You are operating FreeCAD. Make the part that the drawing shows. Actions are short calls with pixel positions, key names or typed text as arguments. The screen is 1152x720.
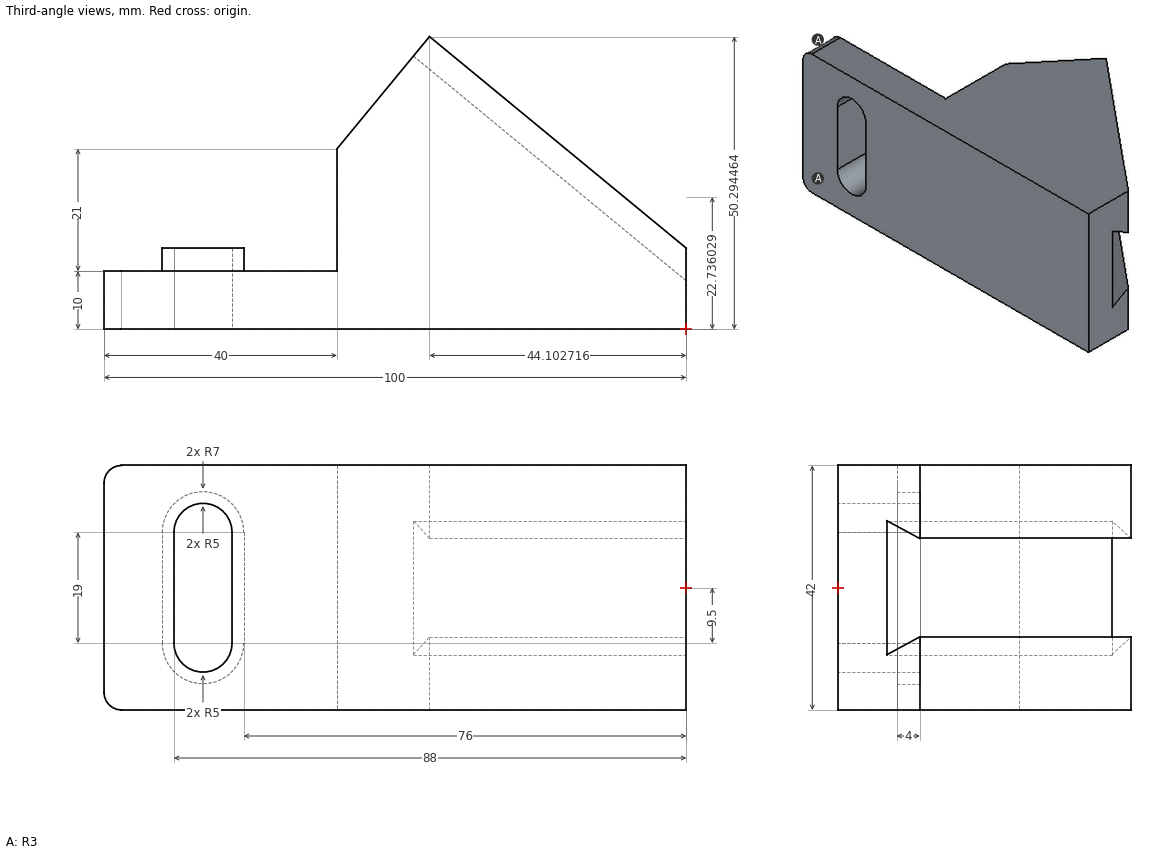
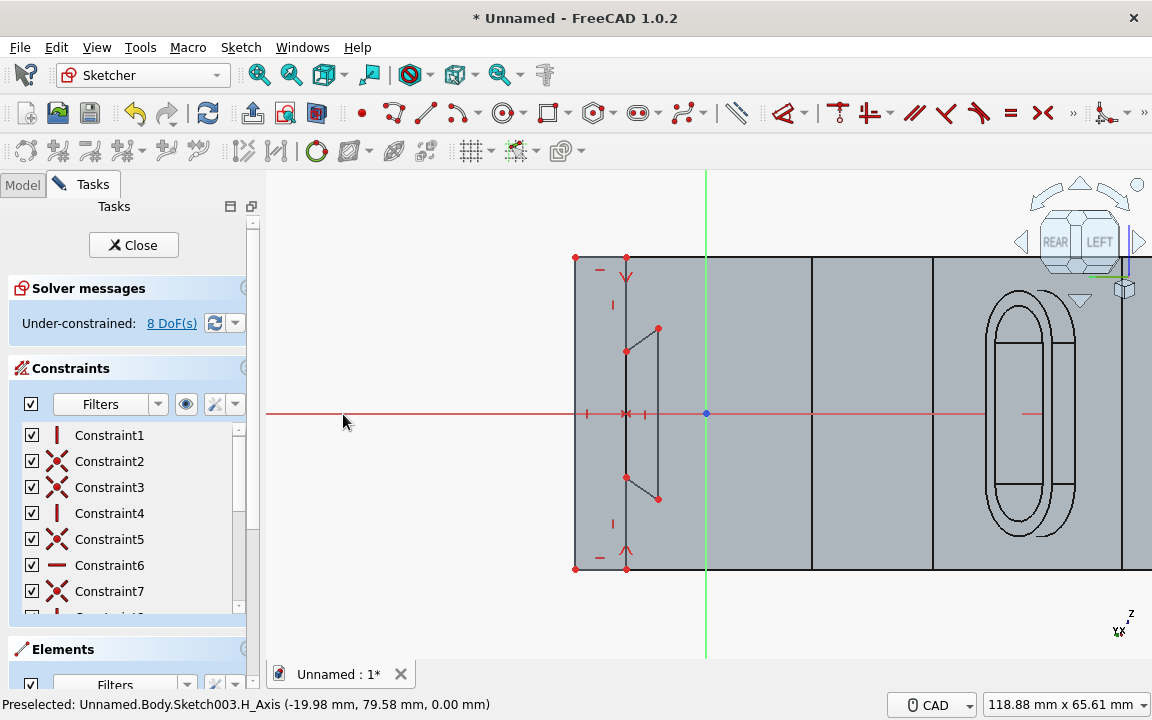
click(658, 449)
click(692, 375)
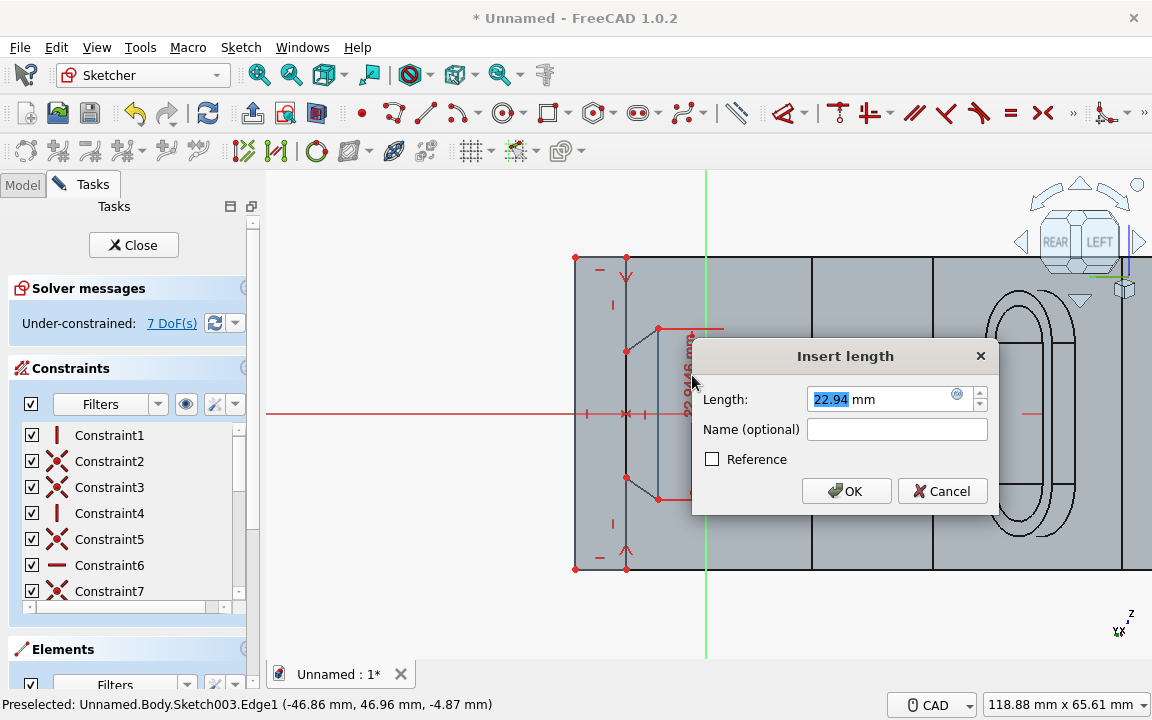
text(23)
key(Return)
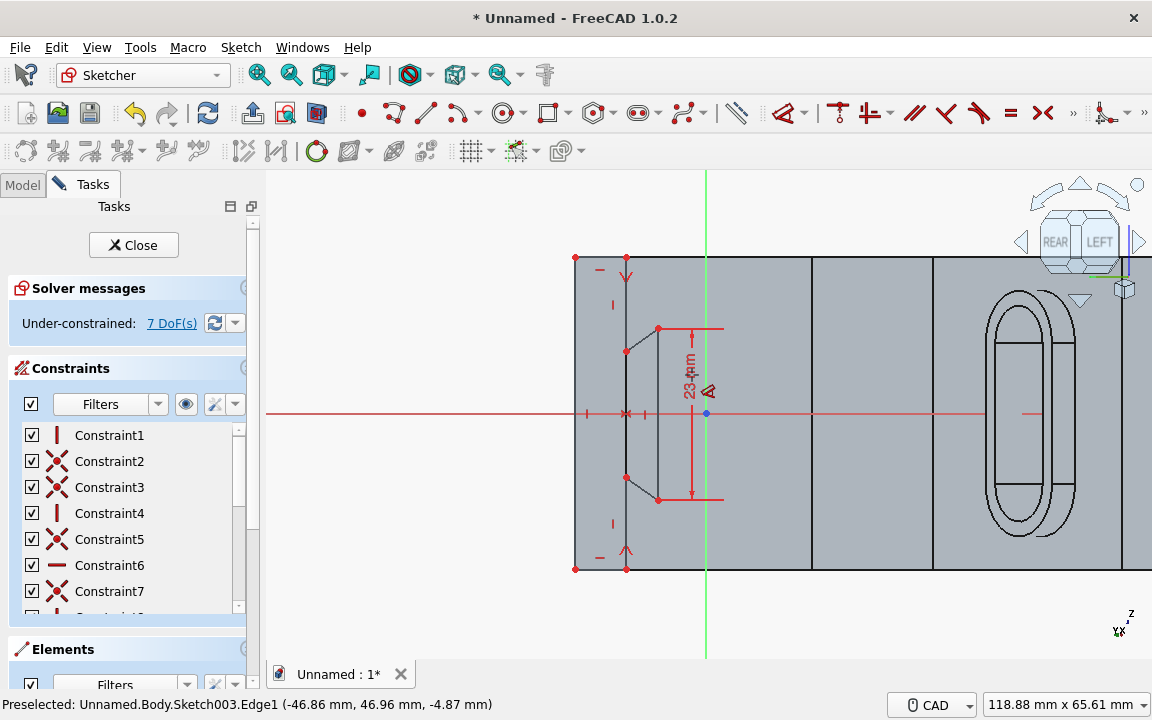
click(575, 351)
click(541, 342)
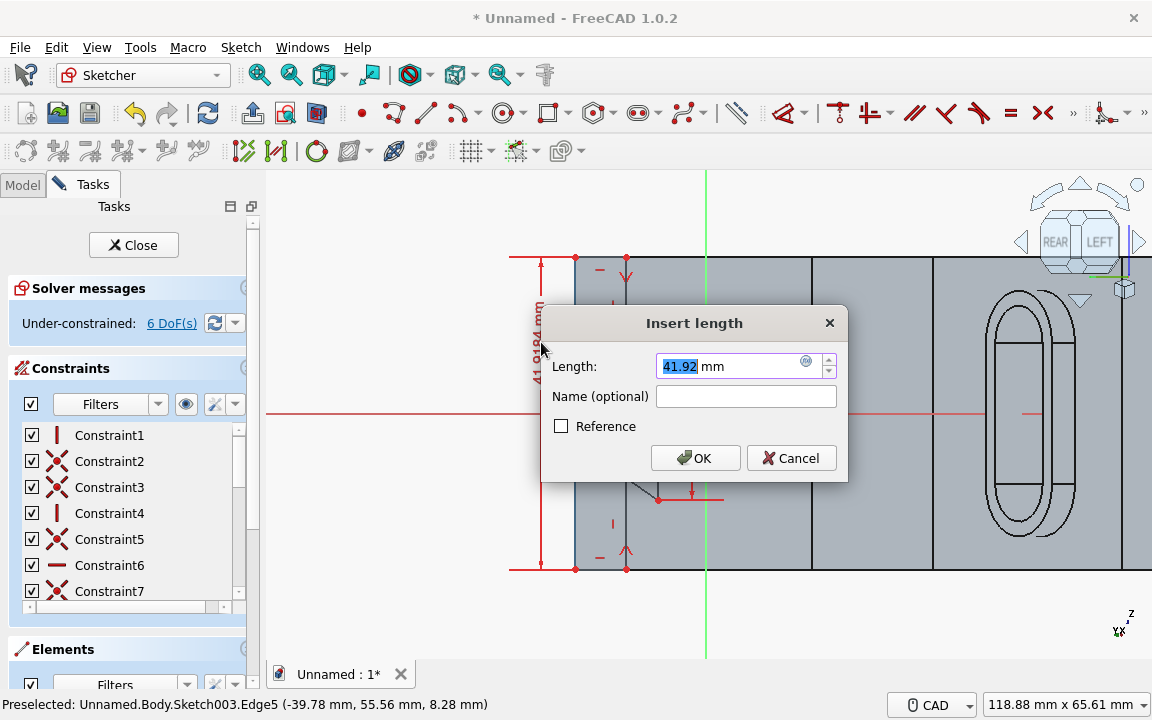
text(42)
key(Return)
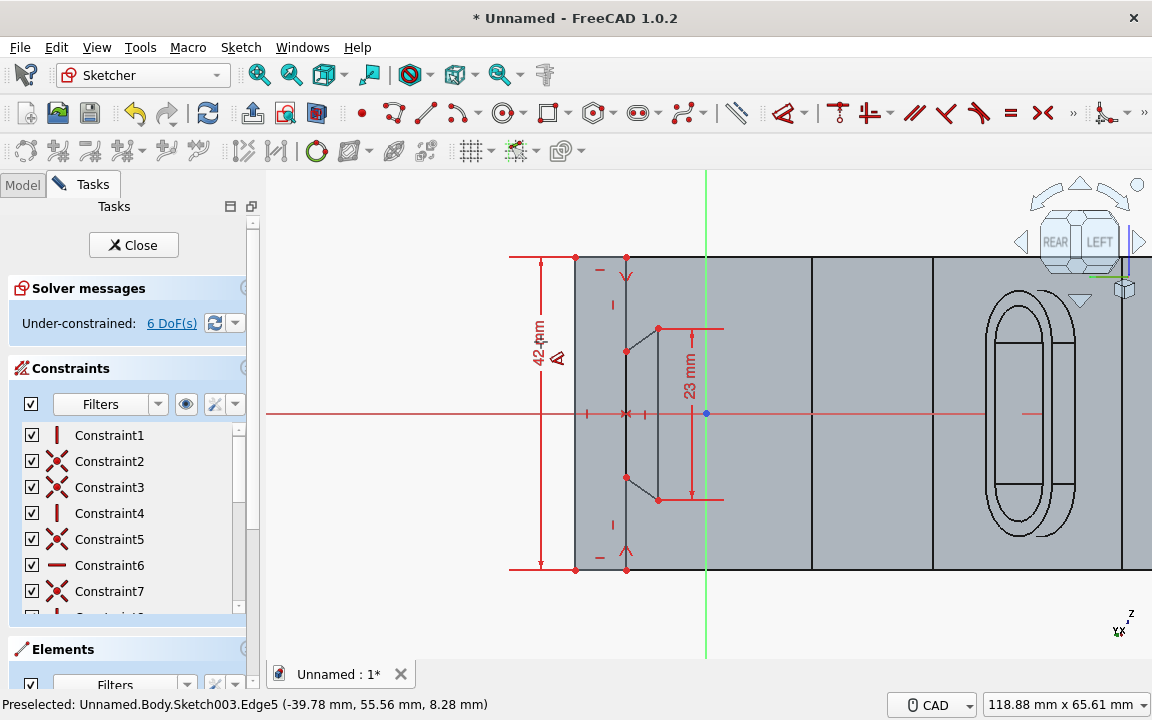
click(658, 500)
click(740, 457)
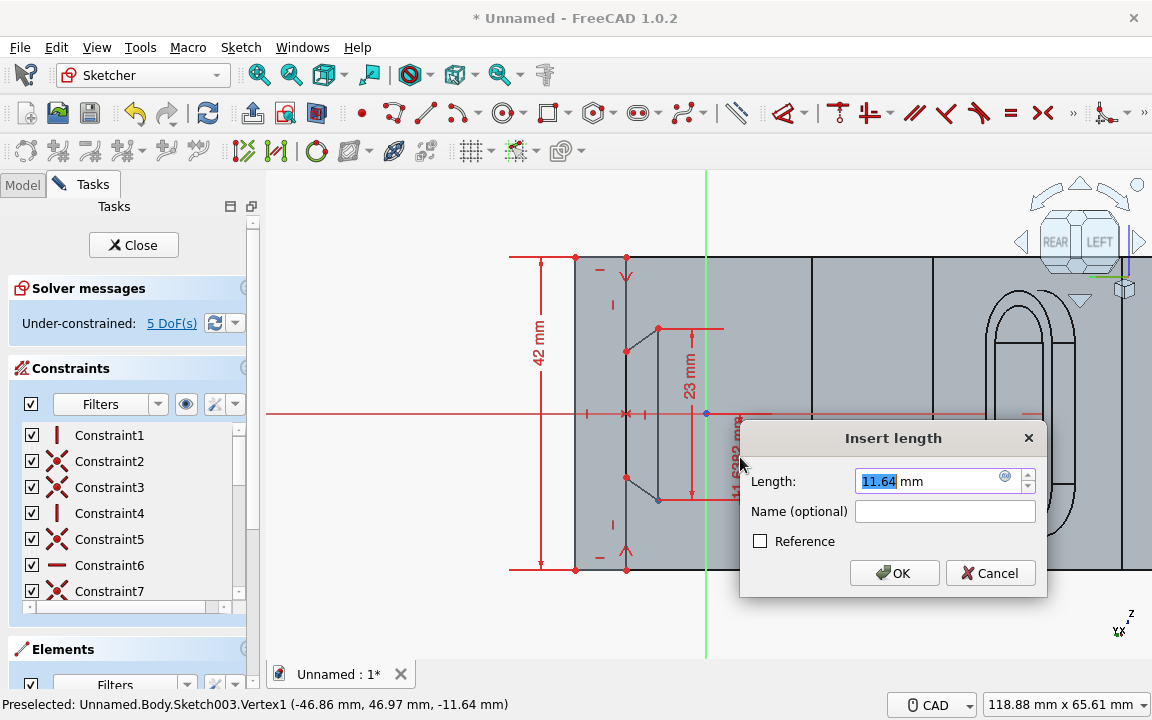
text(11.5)
key(Return)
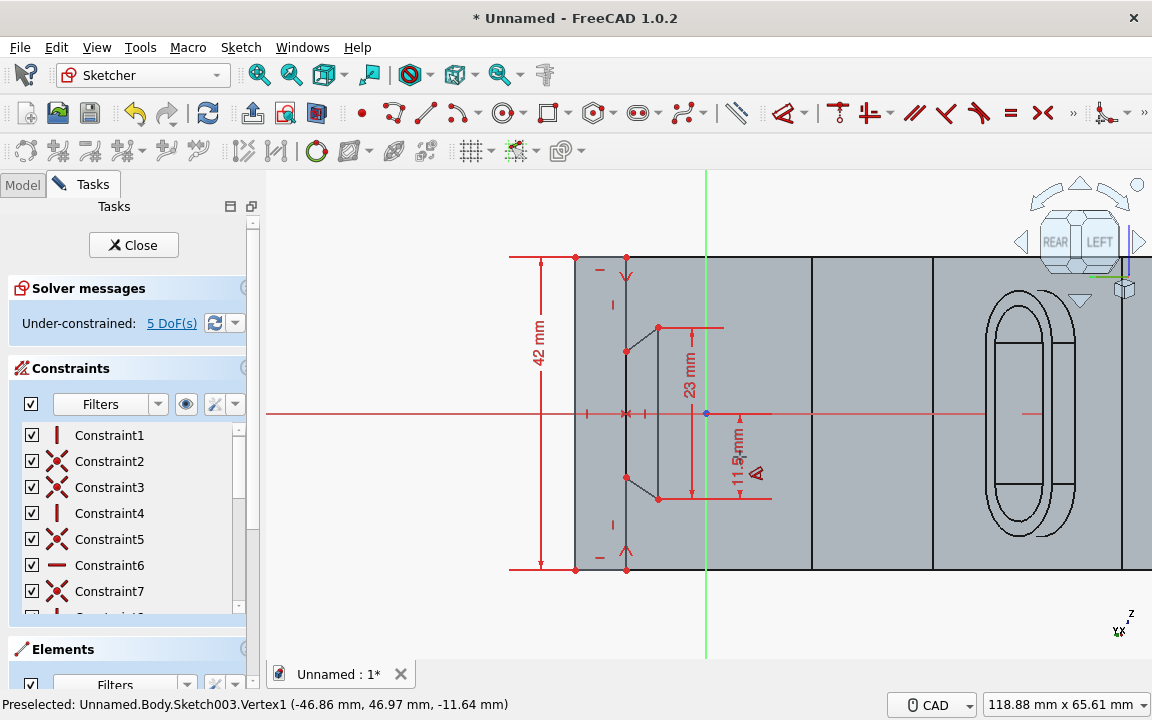
click(611, 257)
click(601, 223)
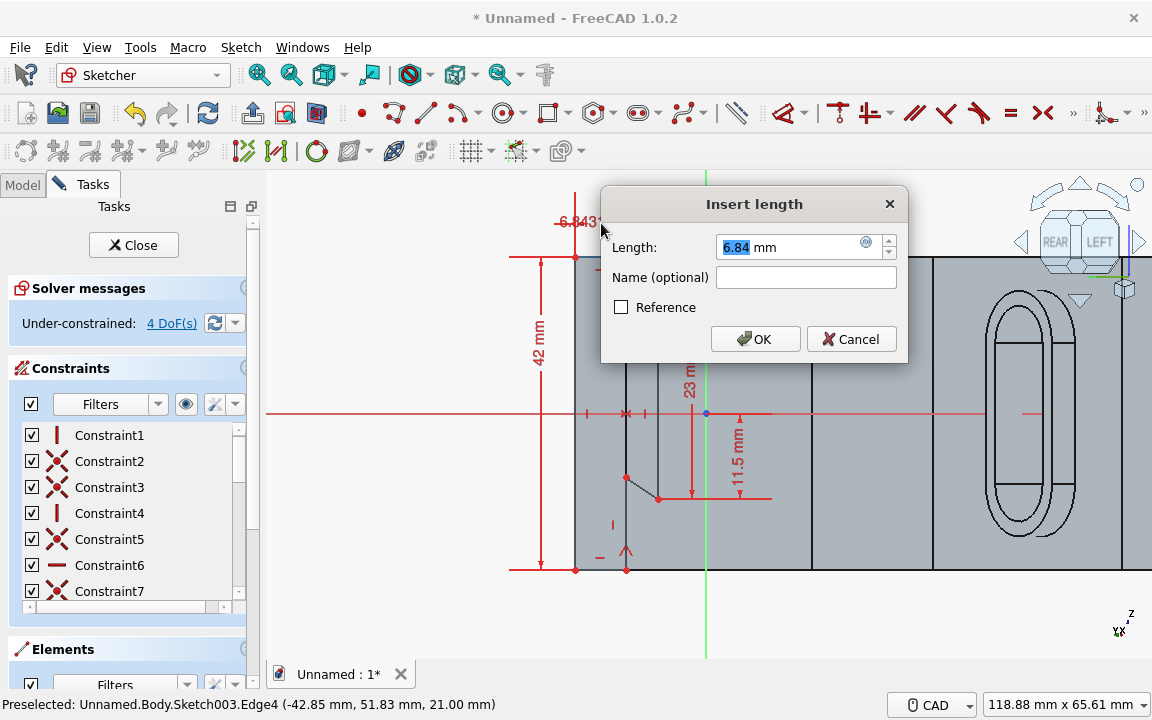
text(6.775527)
key(Return)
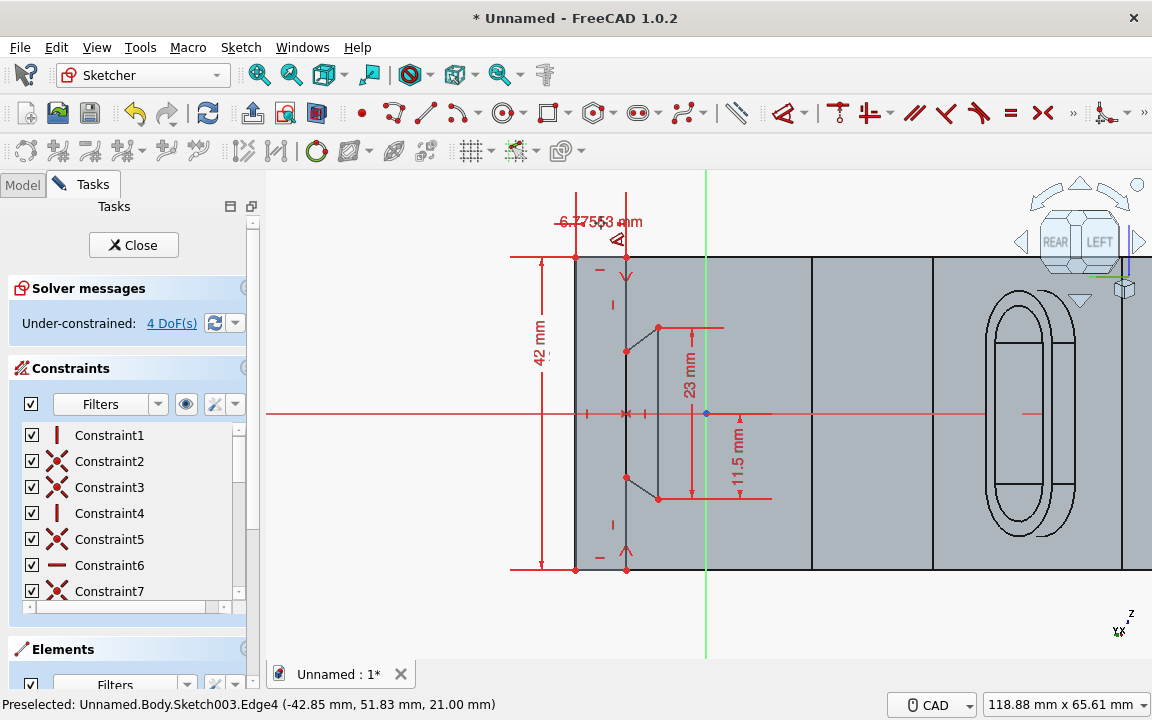
scroll(648, 335, up, 2)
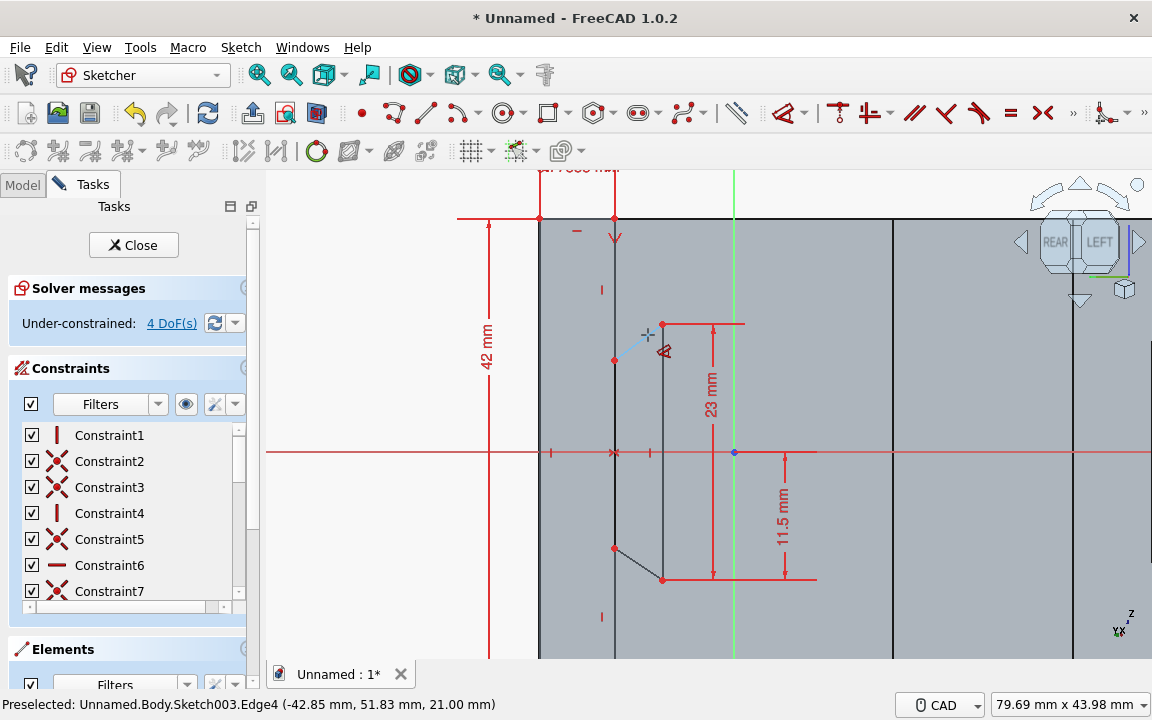
click(648, 335)
click(639, 290)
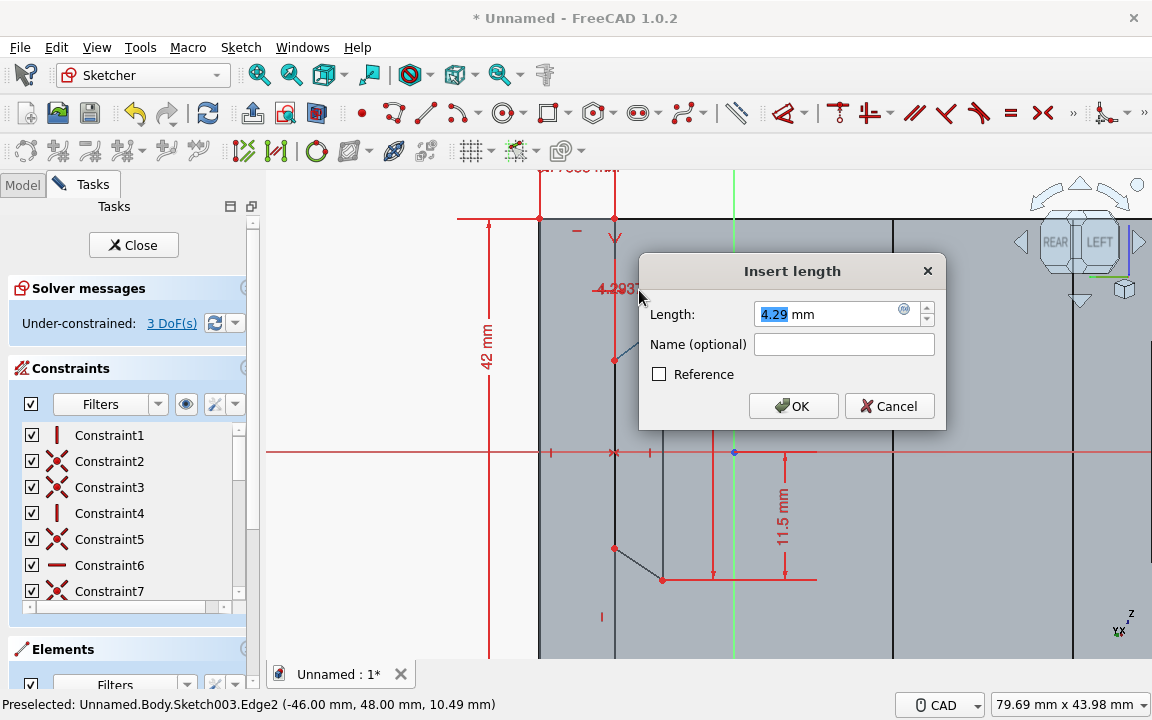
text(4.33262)
key(Return)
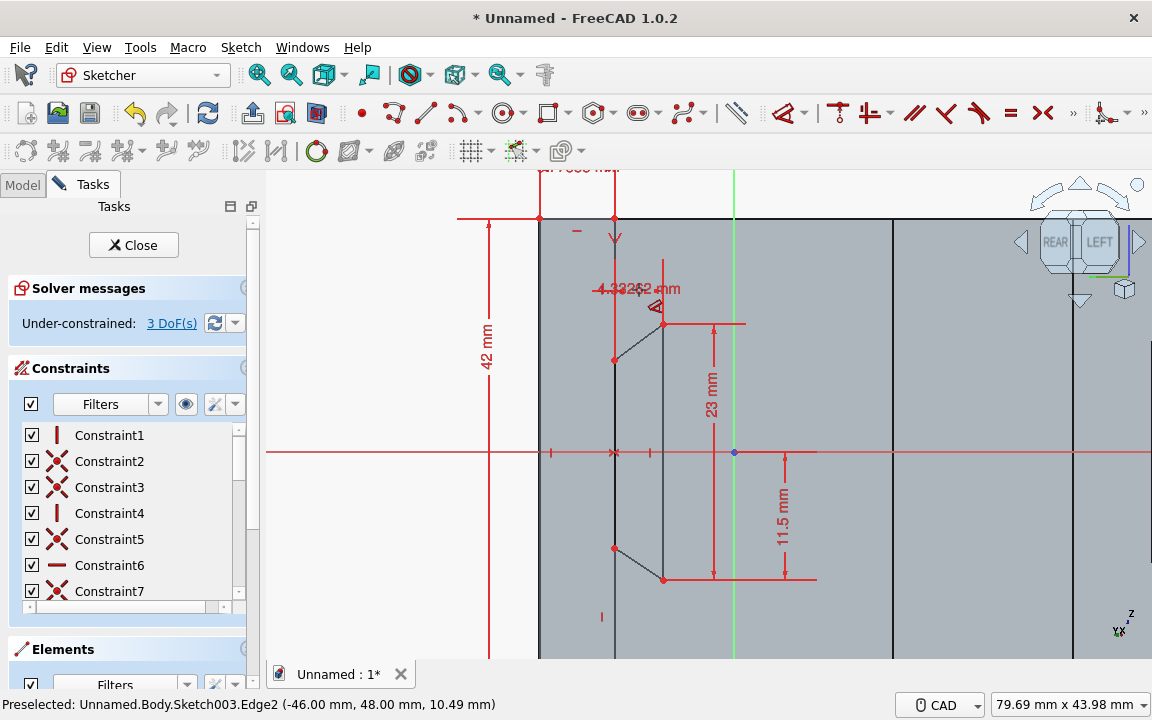
click(615, 318)
click(581, 257)